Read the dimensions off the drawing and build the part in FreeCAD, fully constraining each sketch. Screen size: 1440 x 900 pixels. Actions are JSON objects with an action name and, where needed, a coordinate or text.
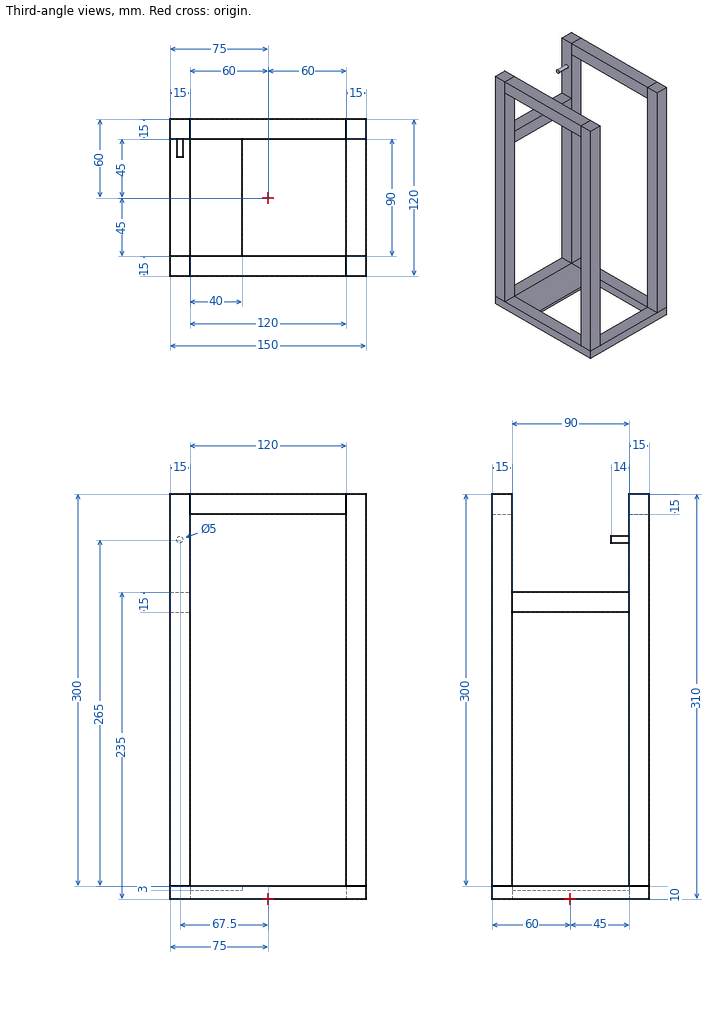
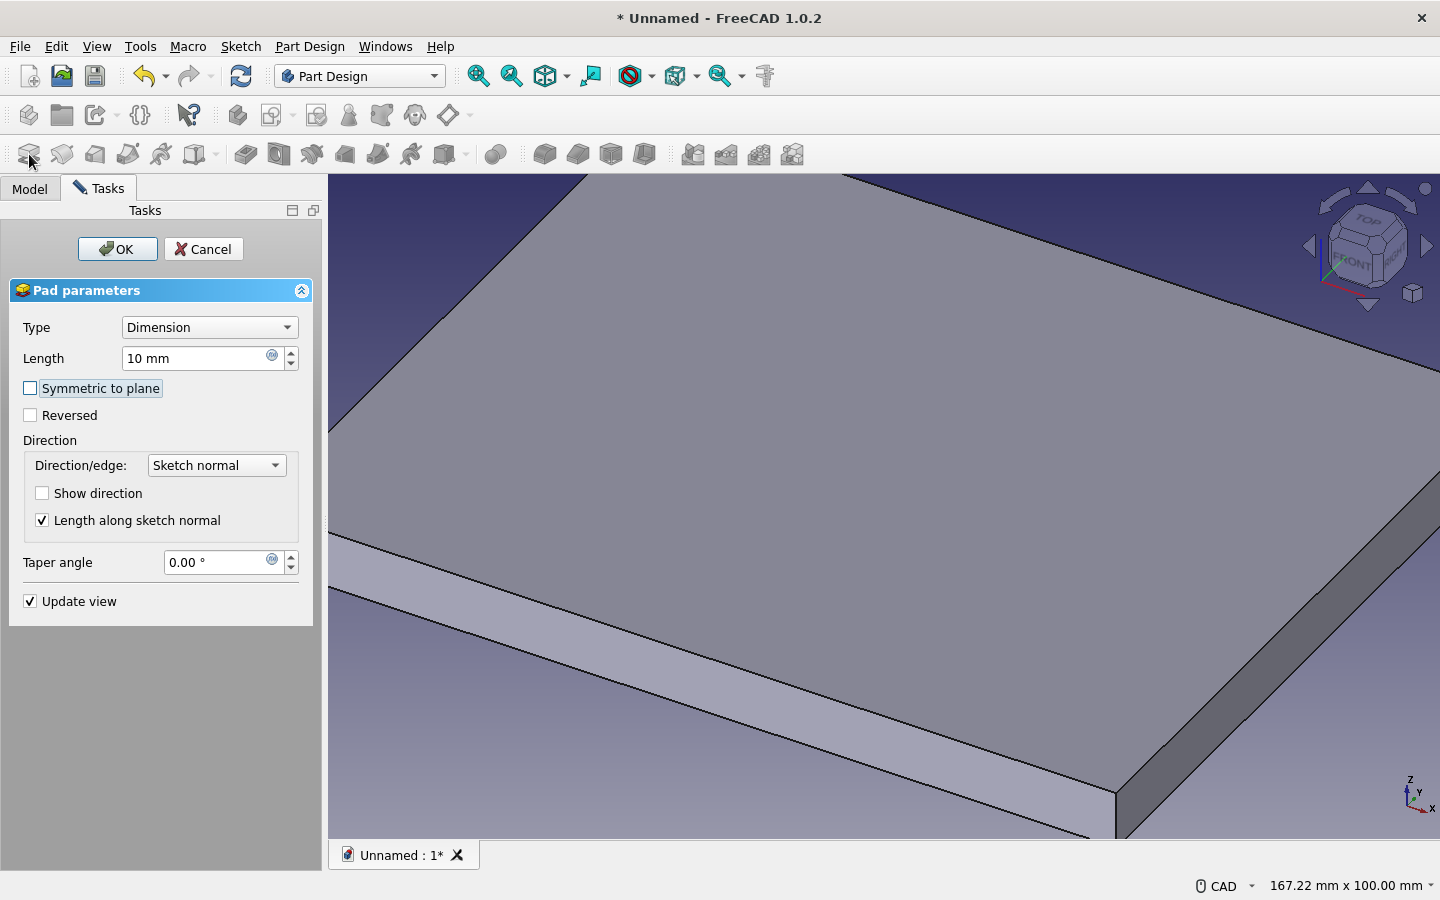
{"action": "left_click", "coordinate": [118, 249]}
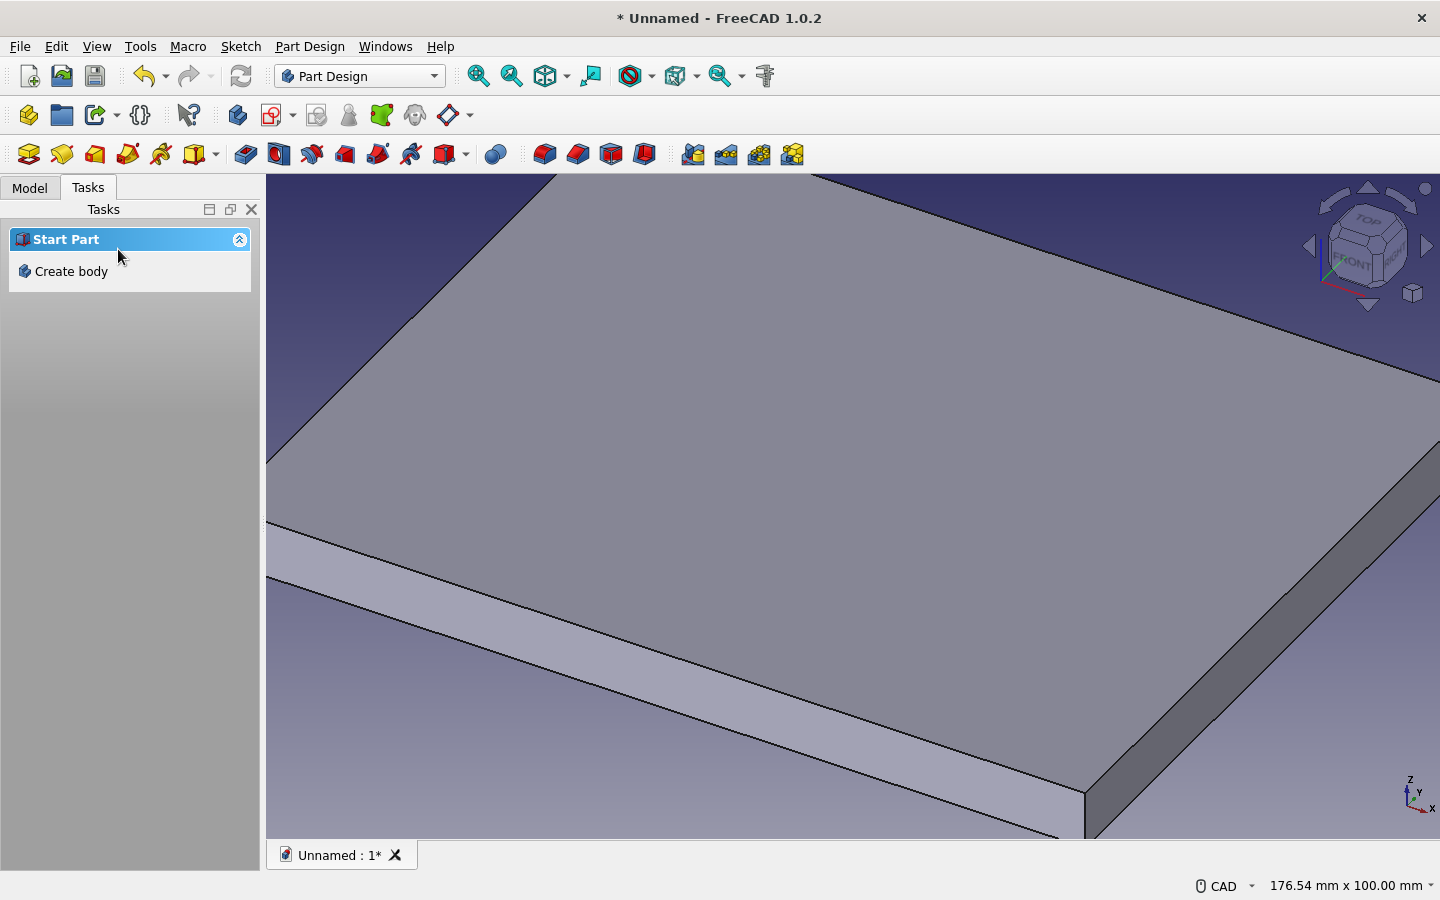
{"action": "left_click", "coordinate": [479, 76]}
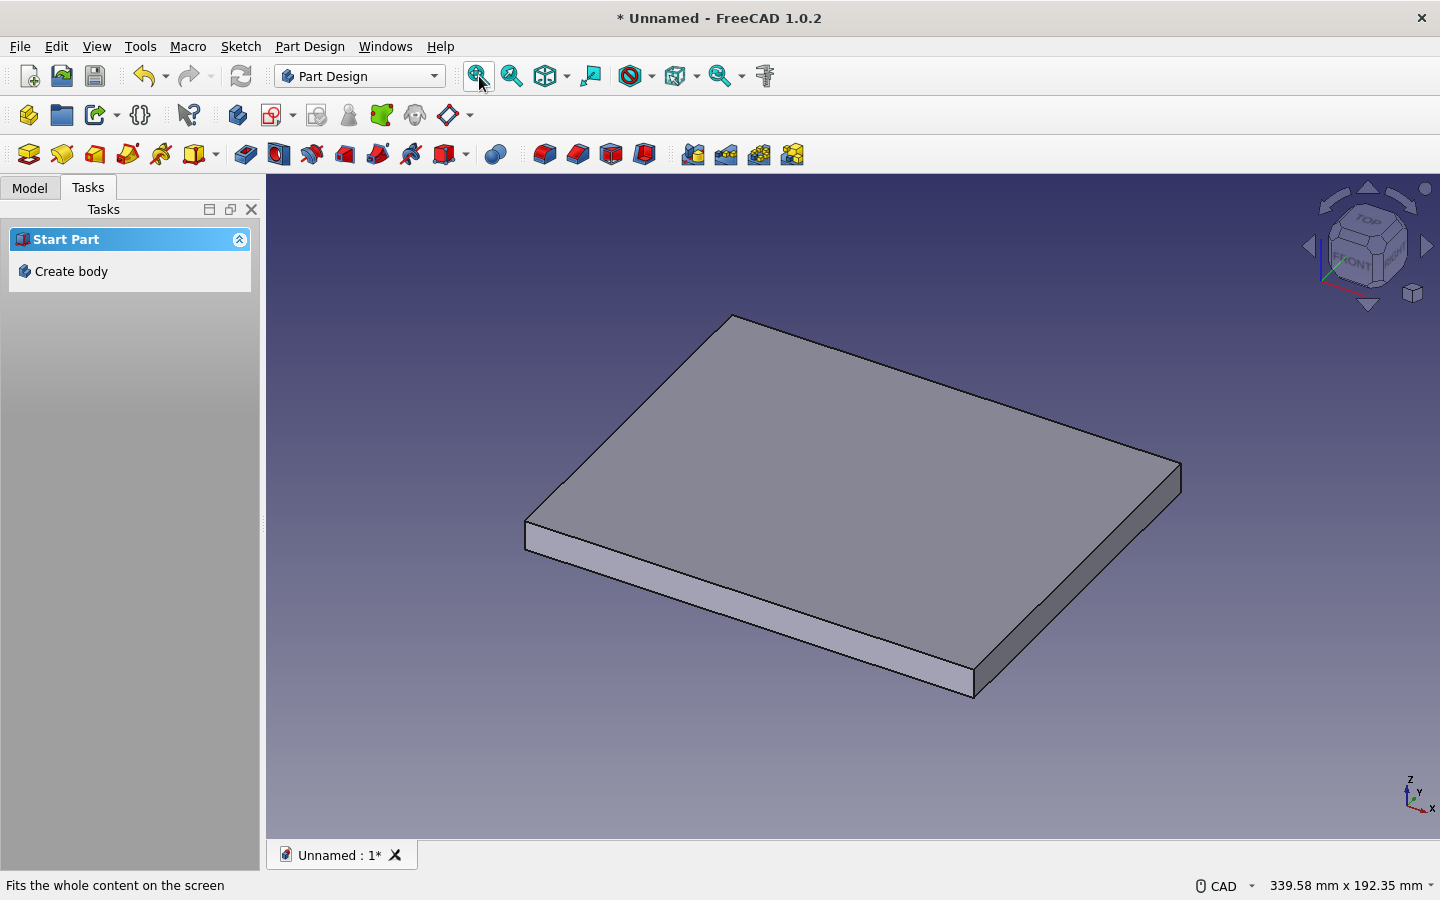
{"action": "left_click", "coordinate": [853, 491]}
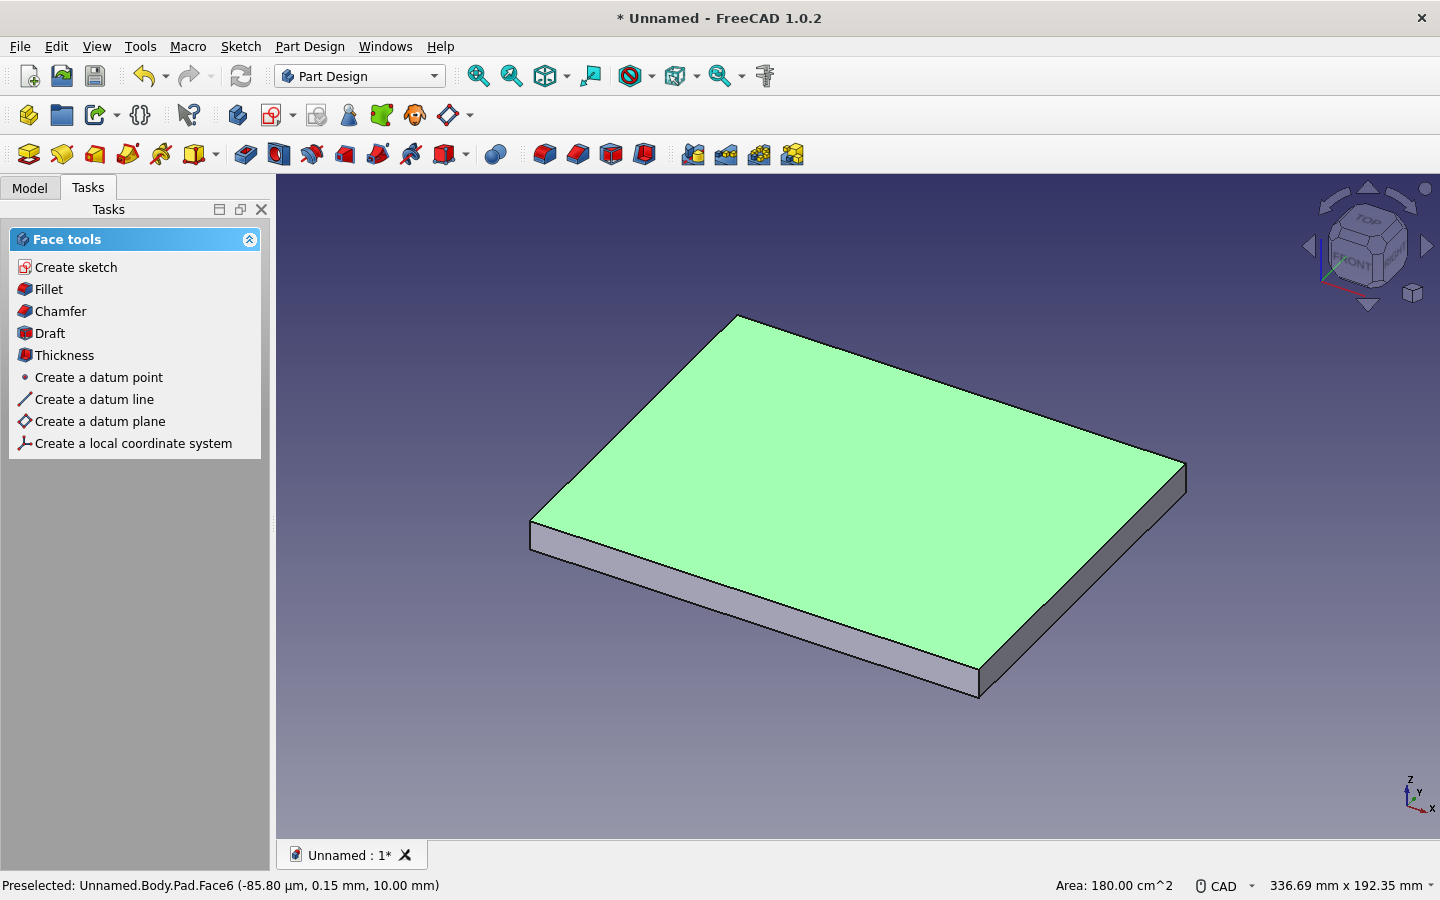
{"action": "left_click", "coordinate": [270, 116]}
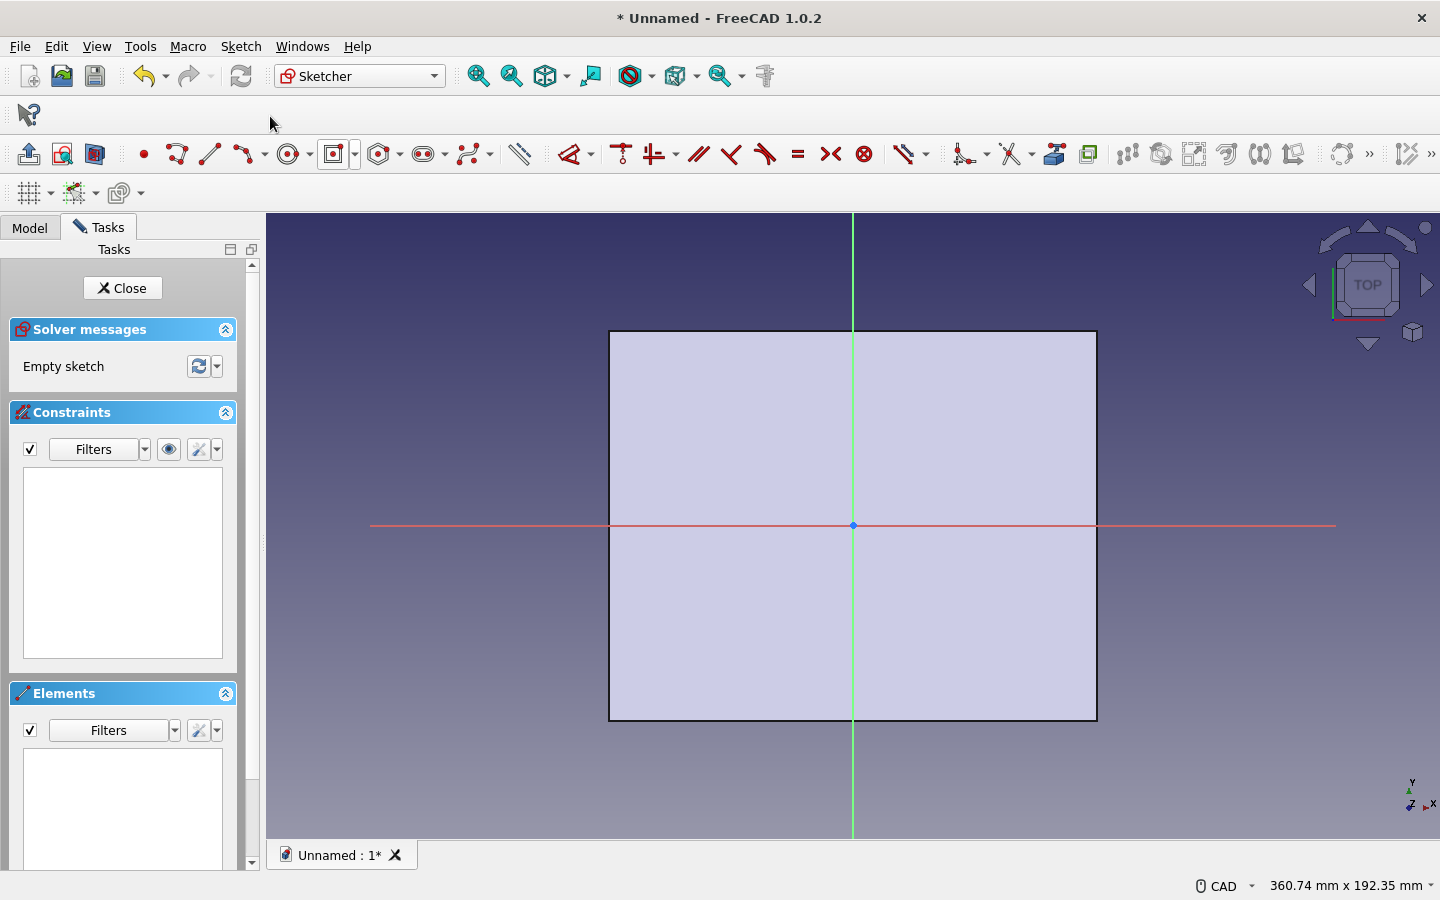
{"action": "scroll", "coordinate": [992, 526], "scroll_direction": "up", "scroll_amount": 2}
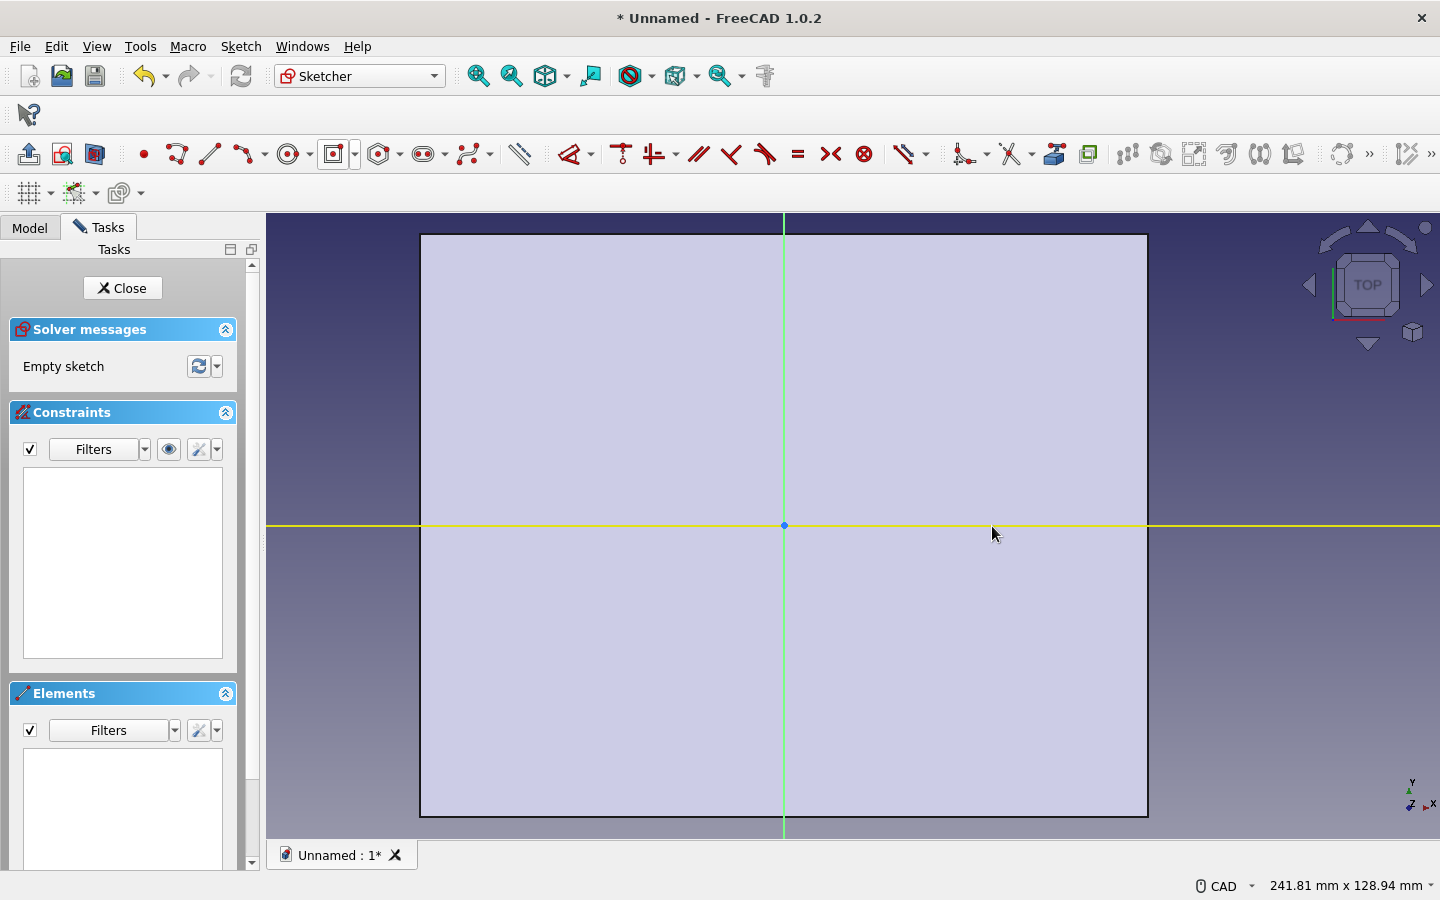
{"action": "left_click", "coordinate": [332, 154]}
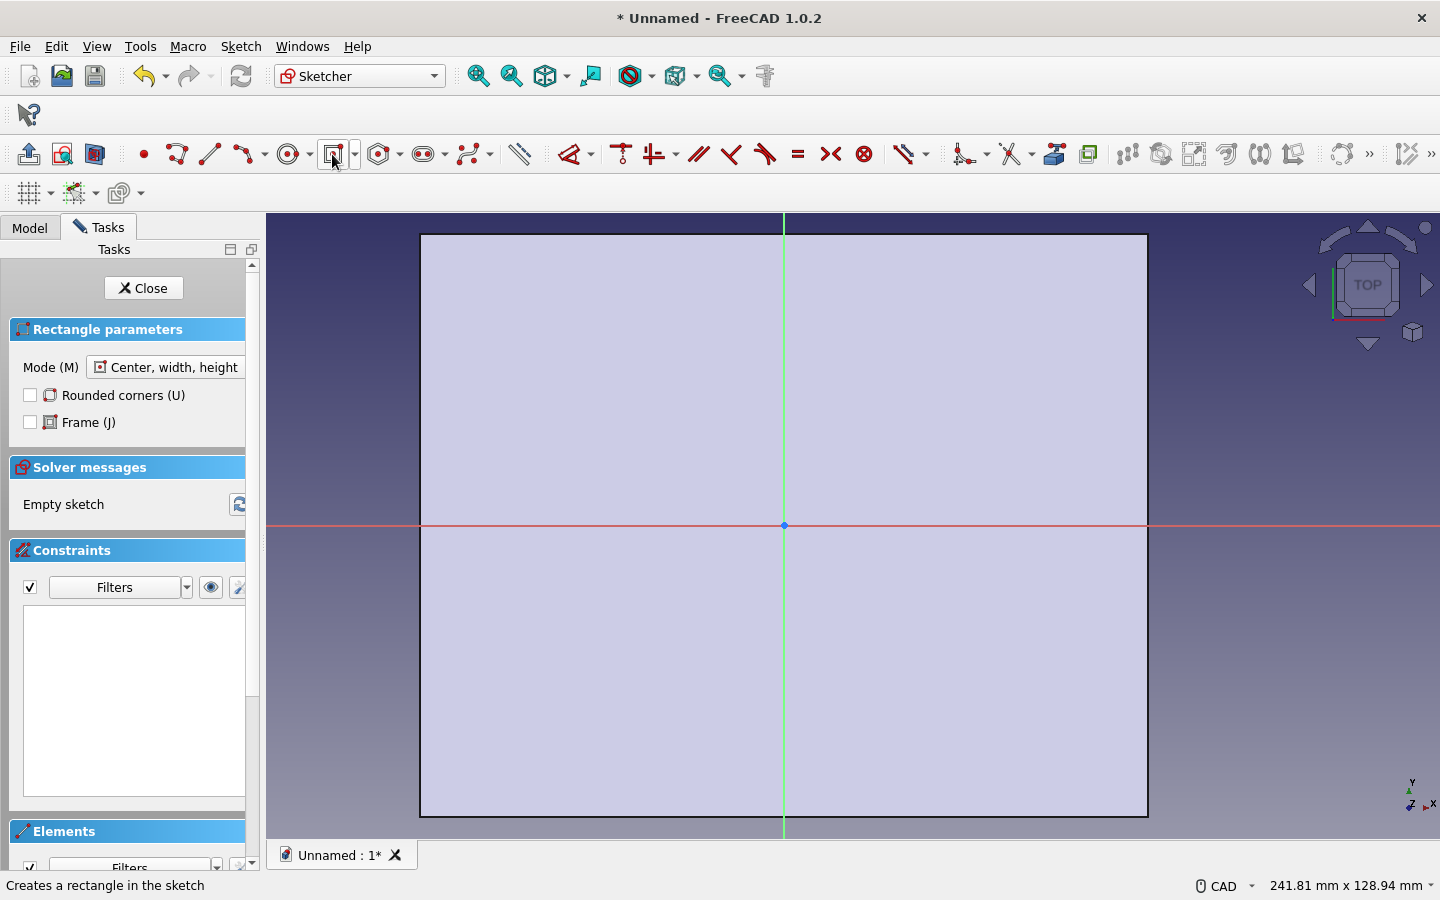
{"action": "left_click", "coordinate": [784, 526]}
{"action": "left_click", "coordinate": [1076, 307]}
{"action": "key", "text": "Escape"}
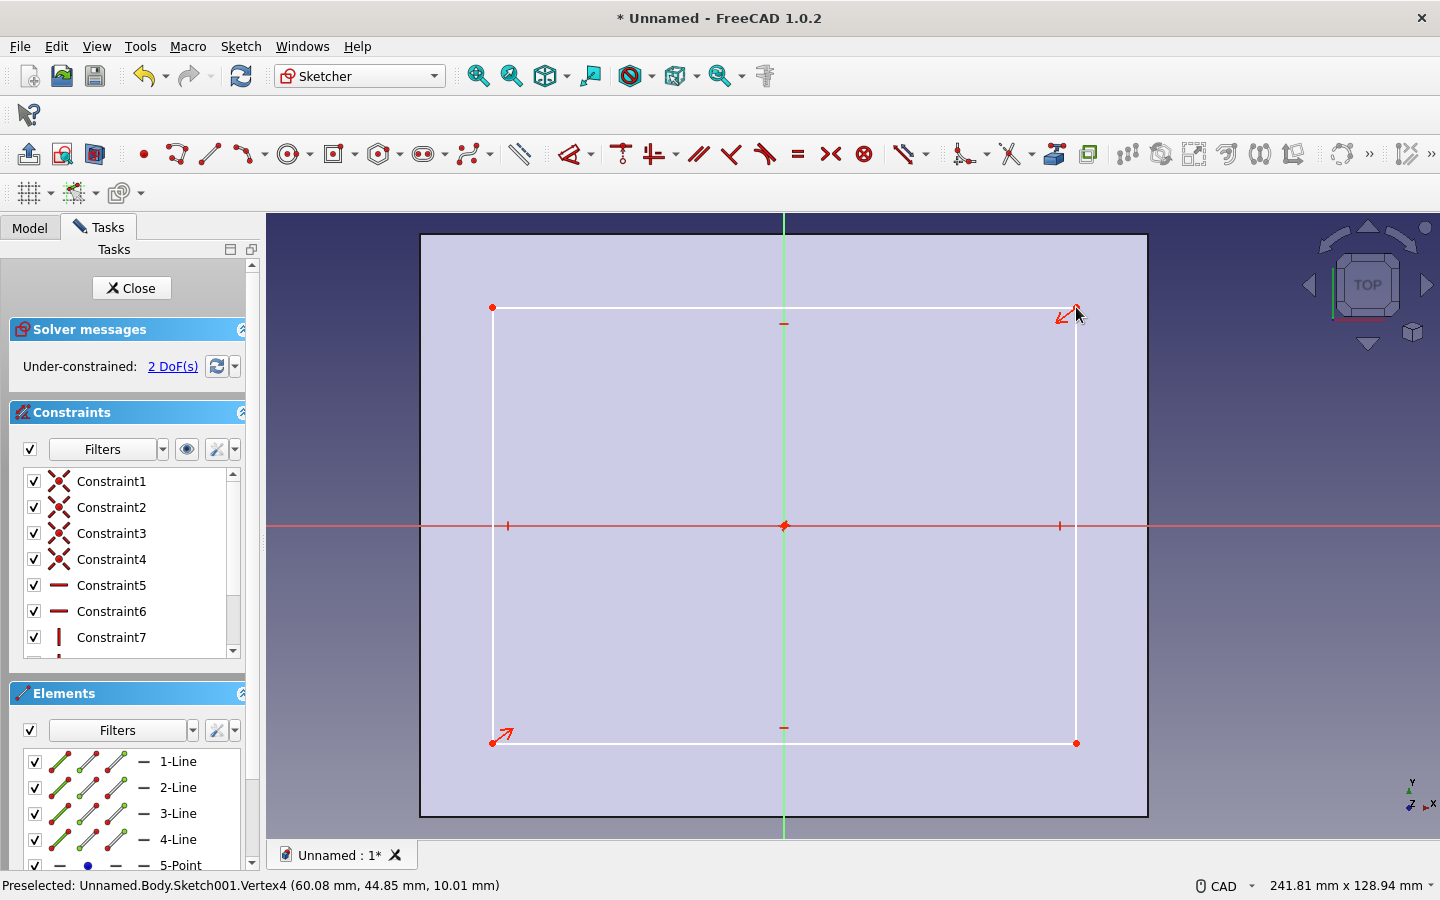
{"action": "left_click", "coordinate": [568, 154]}